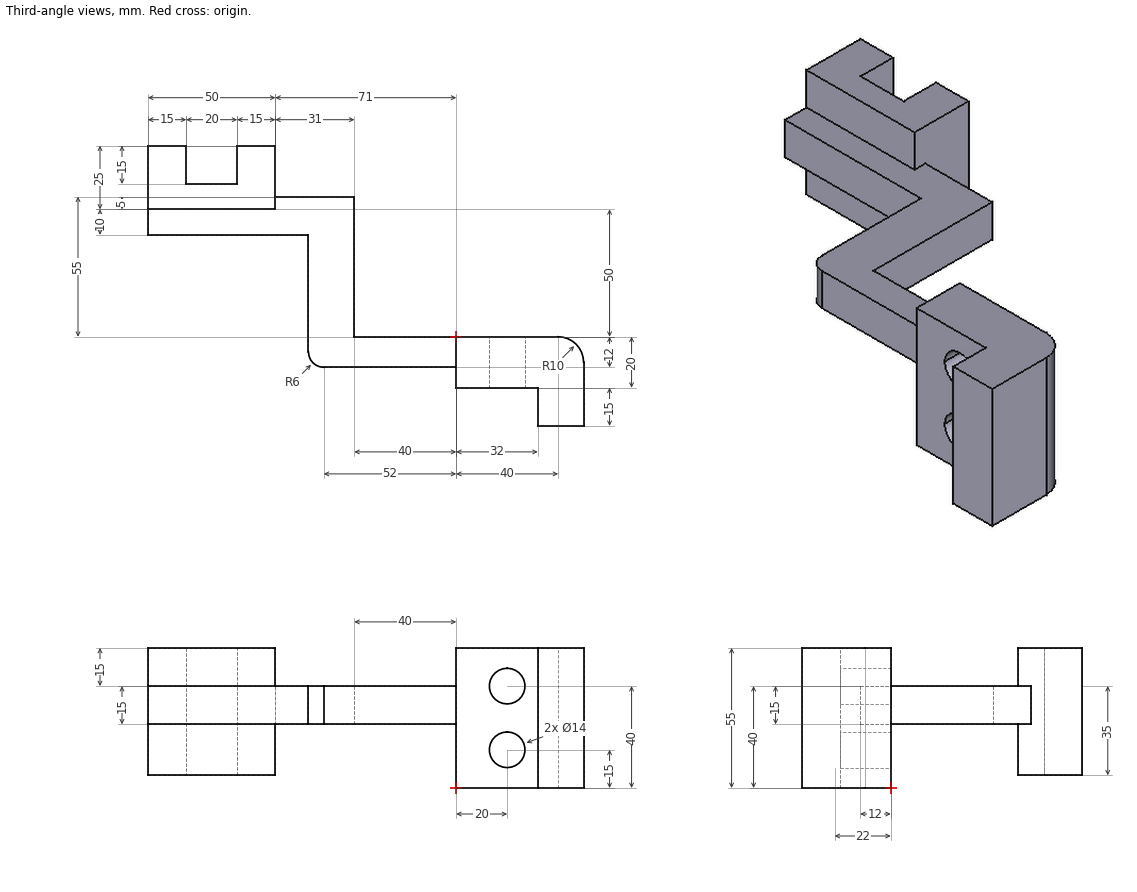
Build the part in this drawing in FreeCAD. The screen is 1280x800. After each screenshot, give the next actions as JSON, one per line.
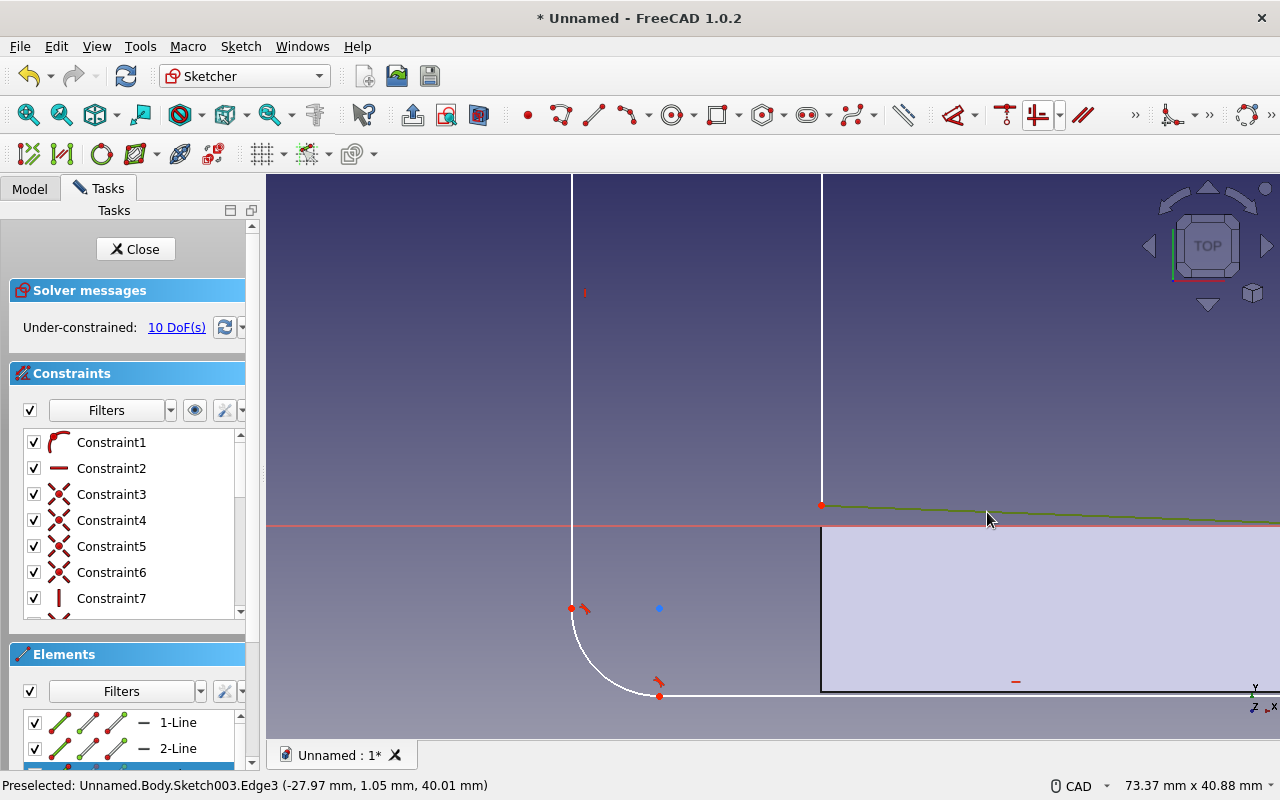
{"action": "left_click", "coordinate": [1060, 116]}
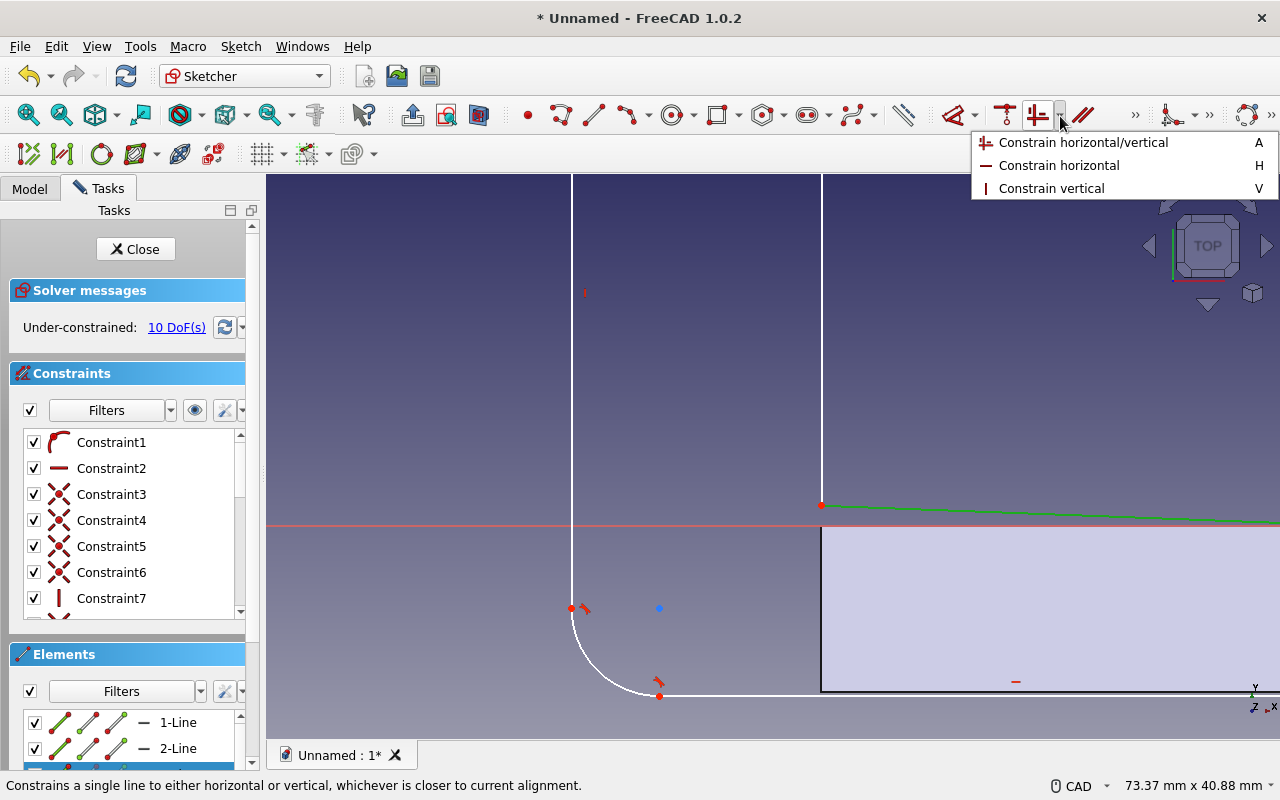
{"action": "left_click", "coordinate": [1125, 166]}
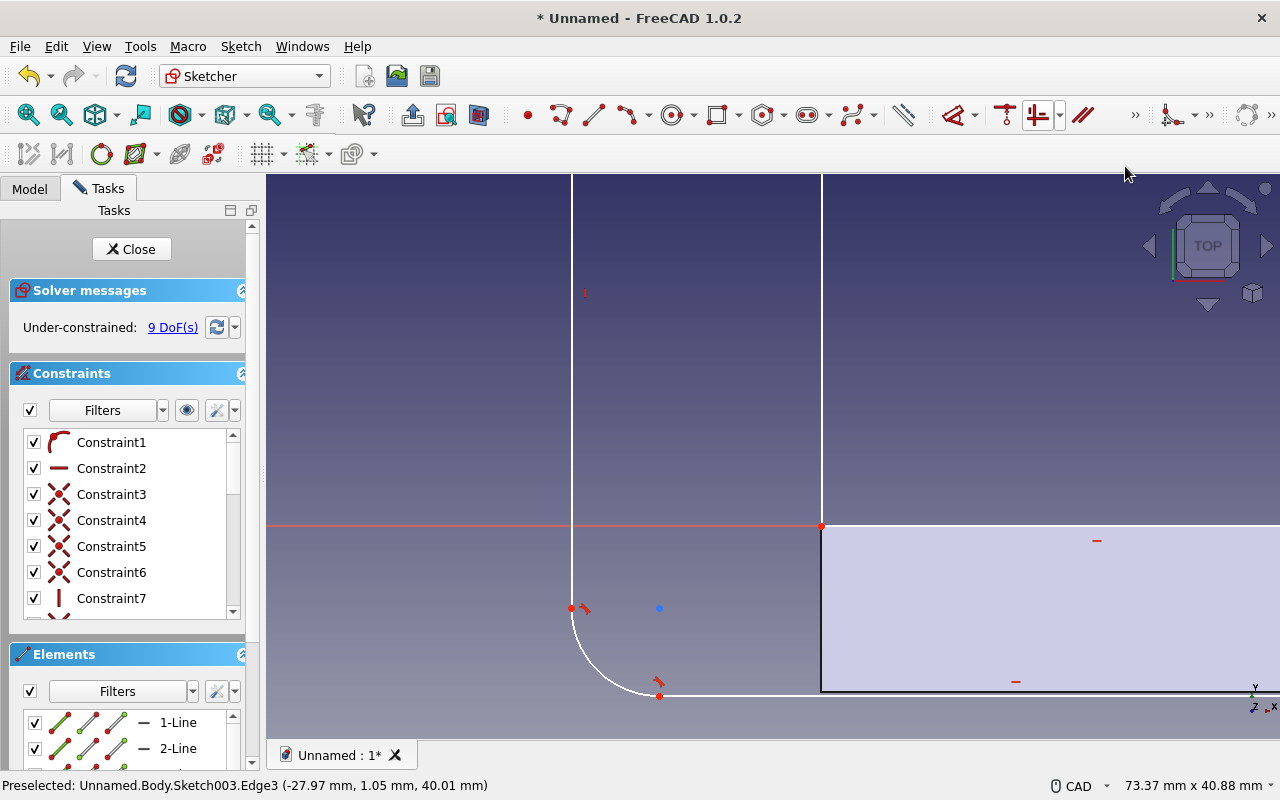
{"action": "left_click", "coordinate": [952, 116]}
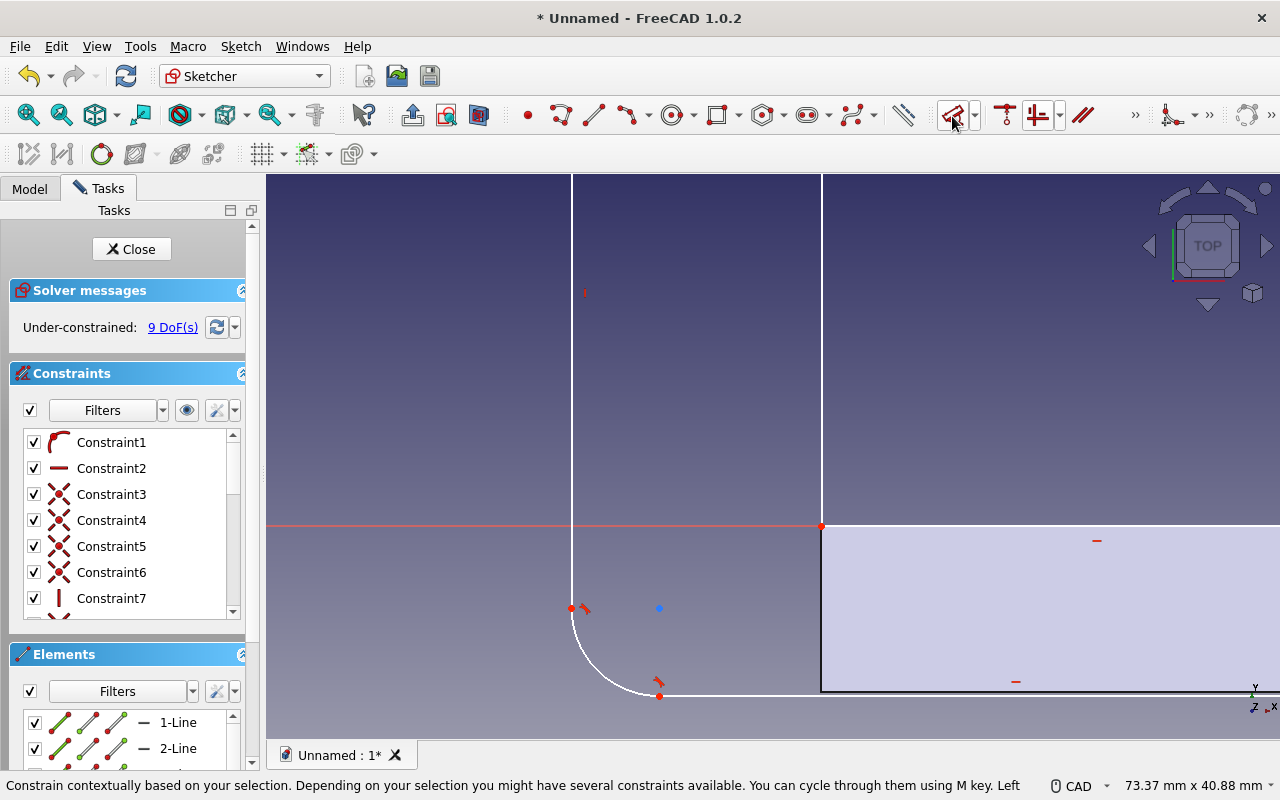
{"action": "left_click", "coordinate": [581, 648]}
{"action": "left_click", "coordinate": [552, 662]}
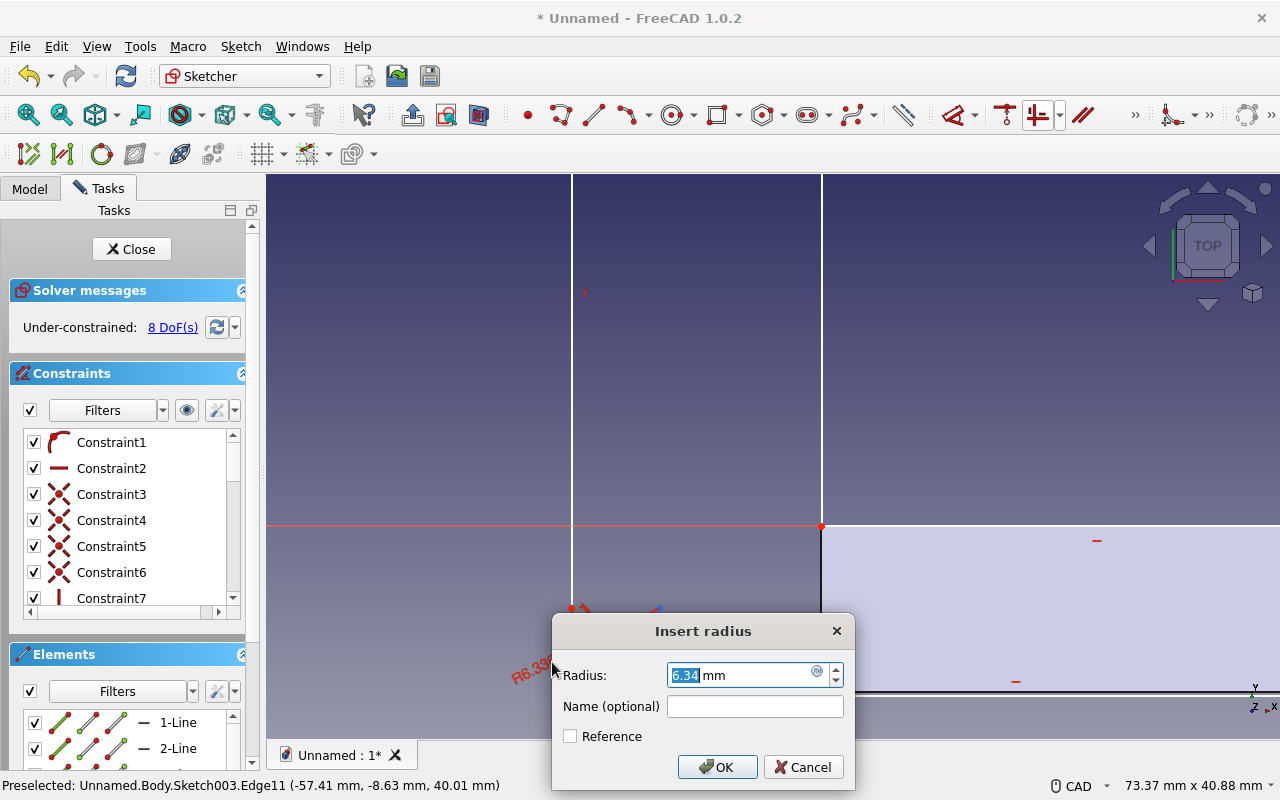
{"action": "type", "text": "6"}
{"action": "key", "text": "Return"}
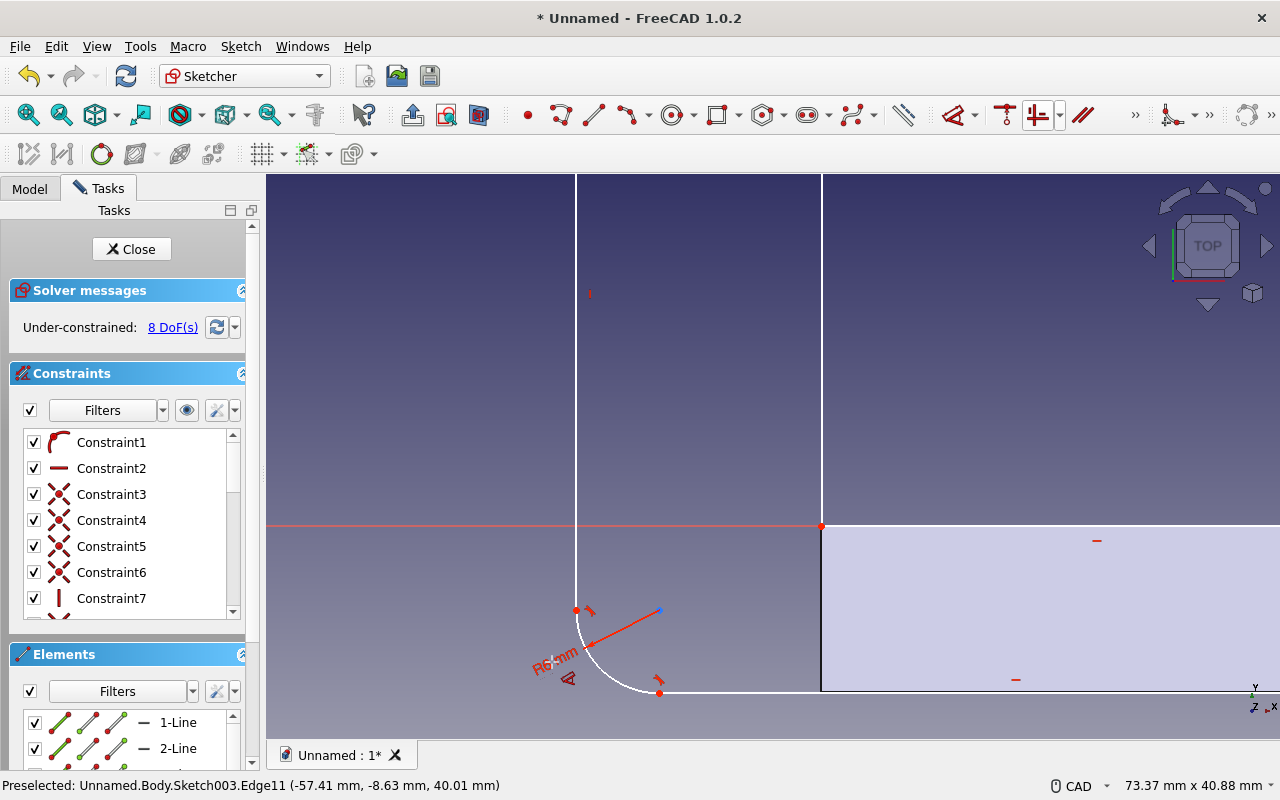
{"action": "scroll", "coordinate": [802, 589], "scroll_direction": "down", "scroll_amount": 5}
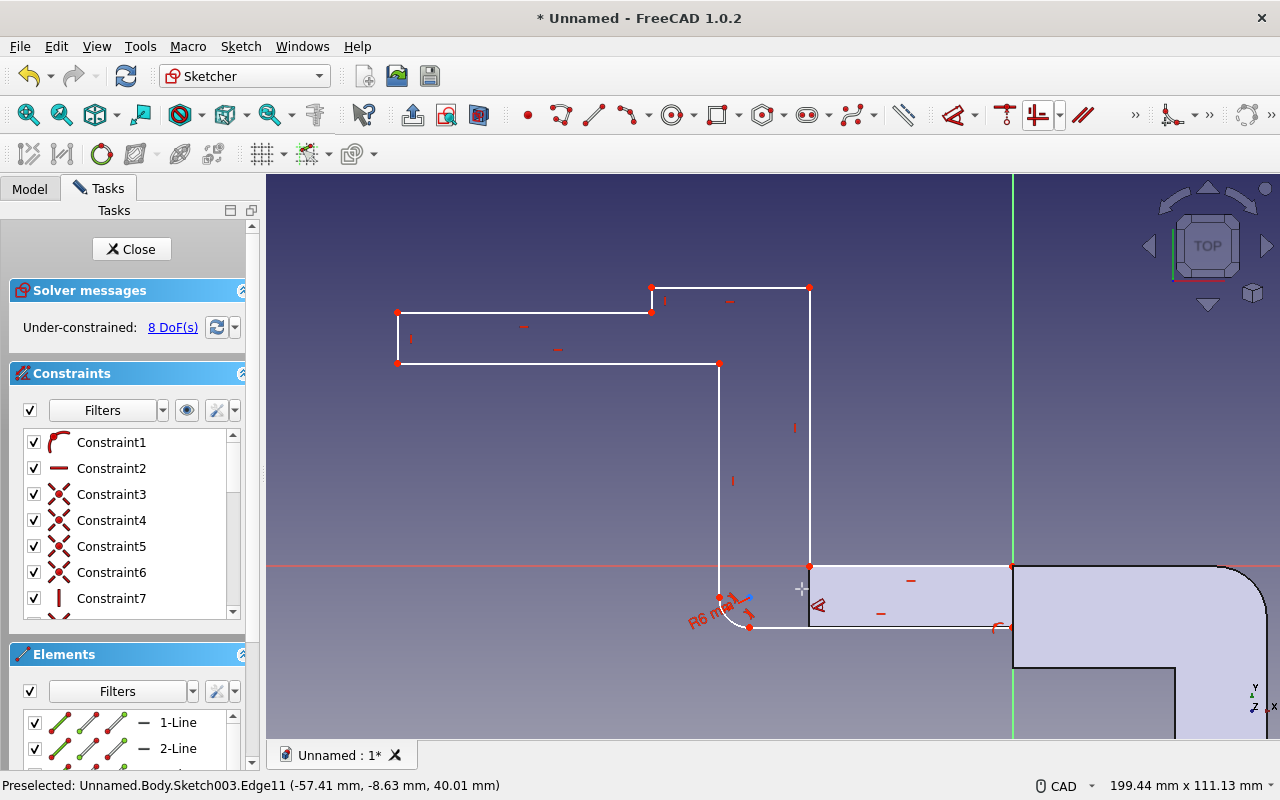
{"action": "scroll", "coordinate": [652, 295], "scroll_direction": "up", "scroll_amount": 4}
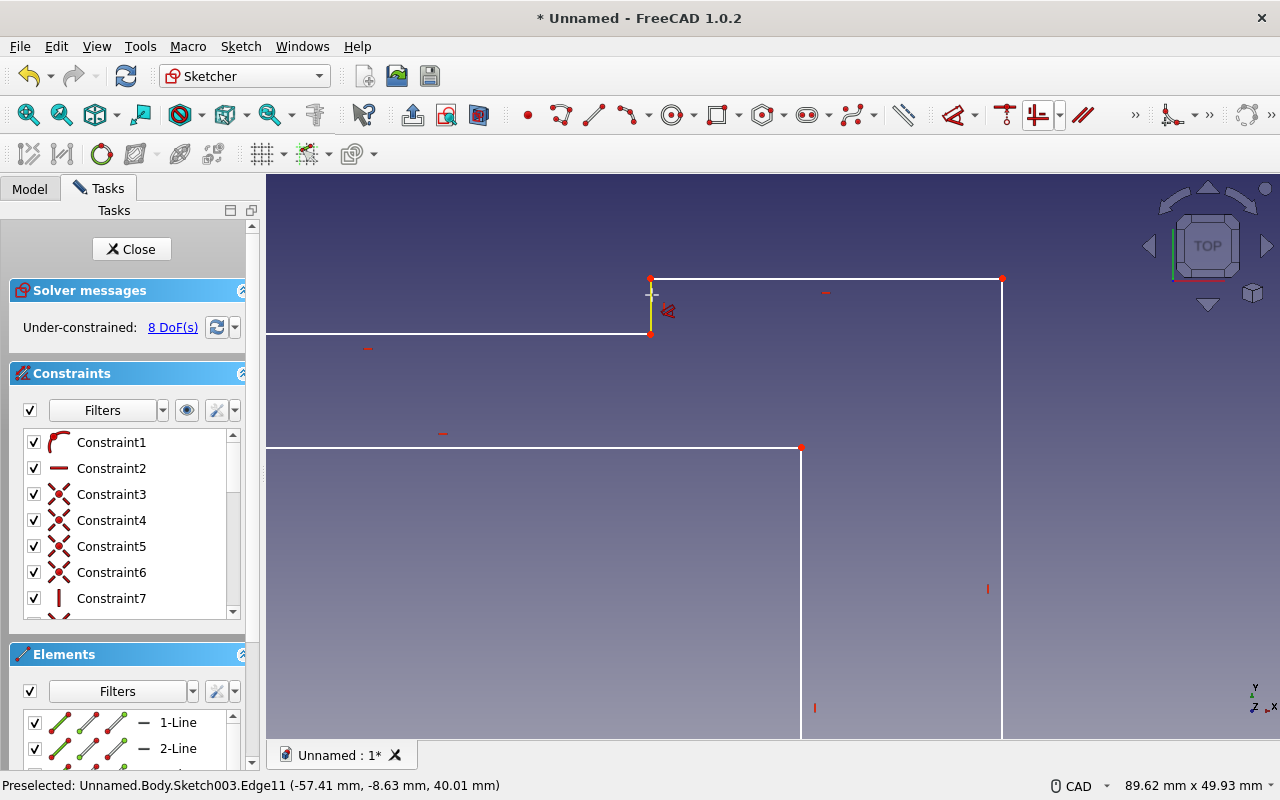
{"action": "left_click", "coordinate": [651, 296]}
{"action": "left_click", "coordinate": [617, 307]}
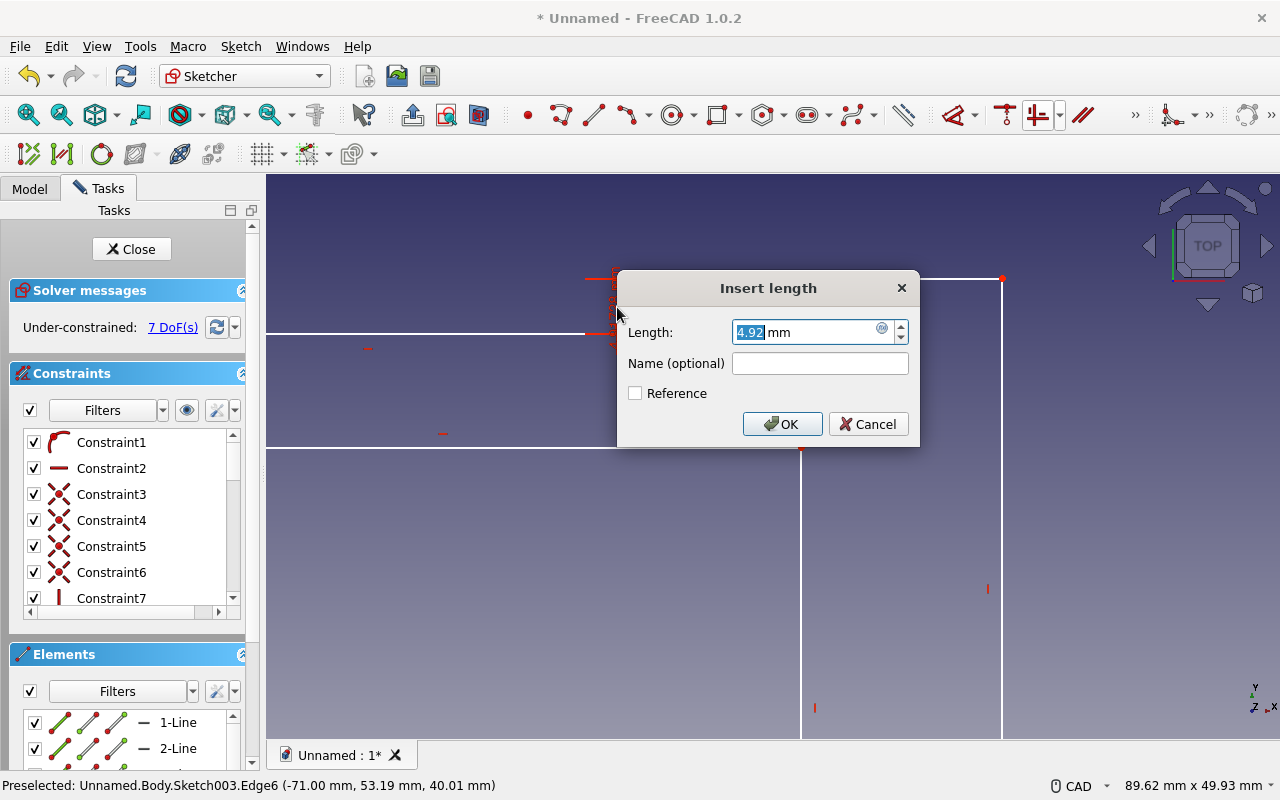
{"action": "type", "text": "5"}
{"action": "key", "text": "Return"}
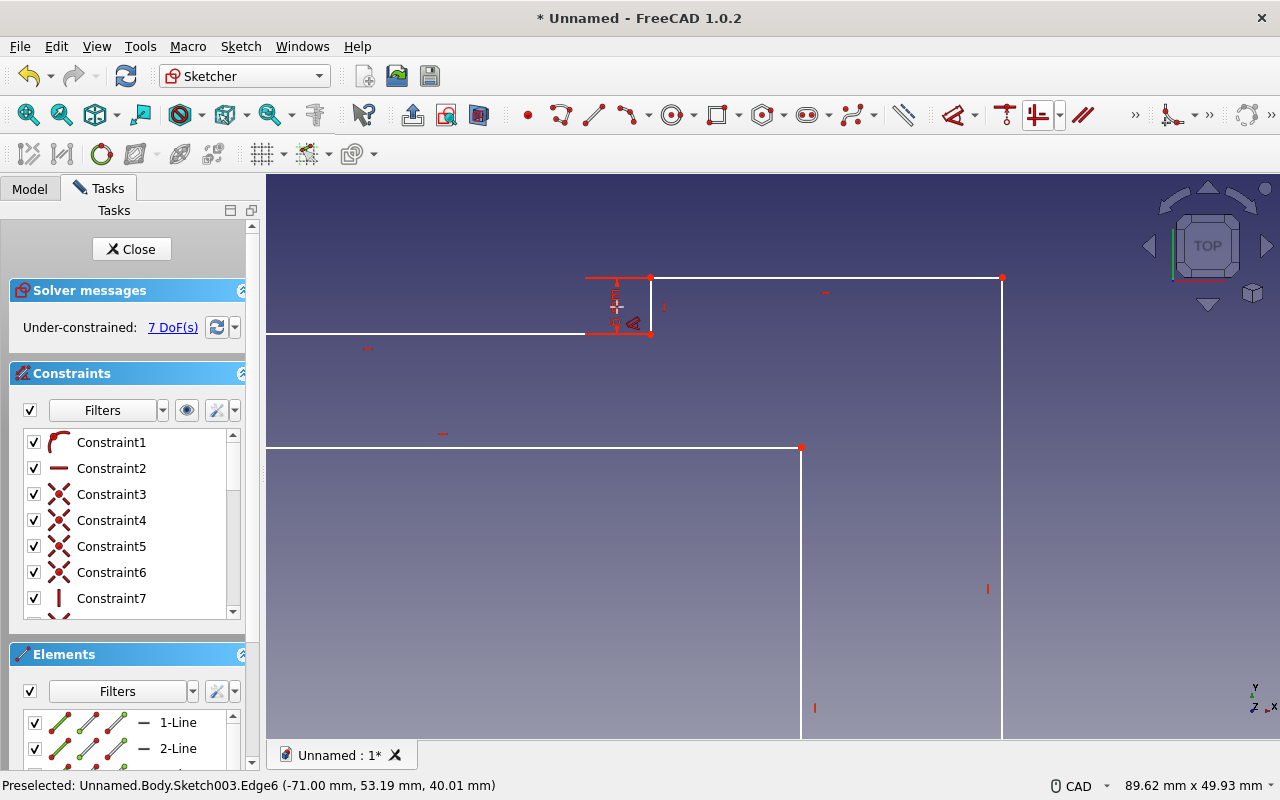
{"action": "scroll", "coordinate": [651, 294], "scroll_direction": "down", "scroll_amount": 4}